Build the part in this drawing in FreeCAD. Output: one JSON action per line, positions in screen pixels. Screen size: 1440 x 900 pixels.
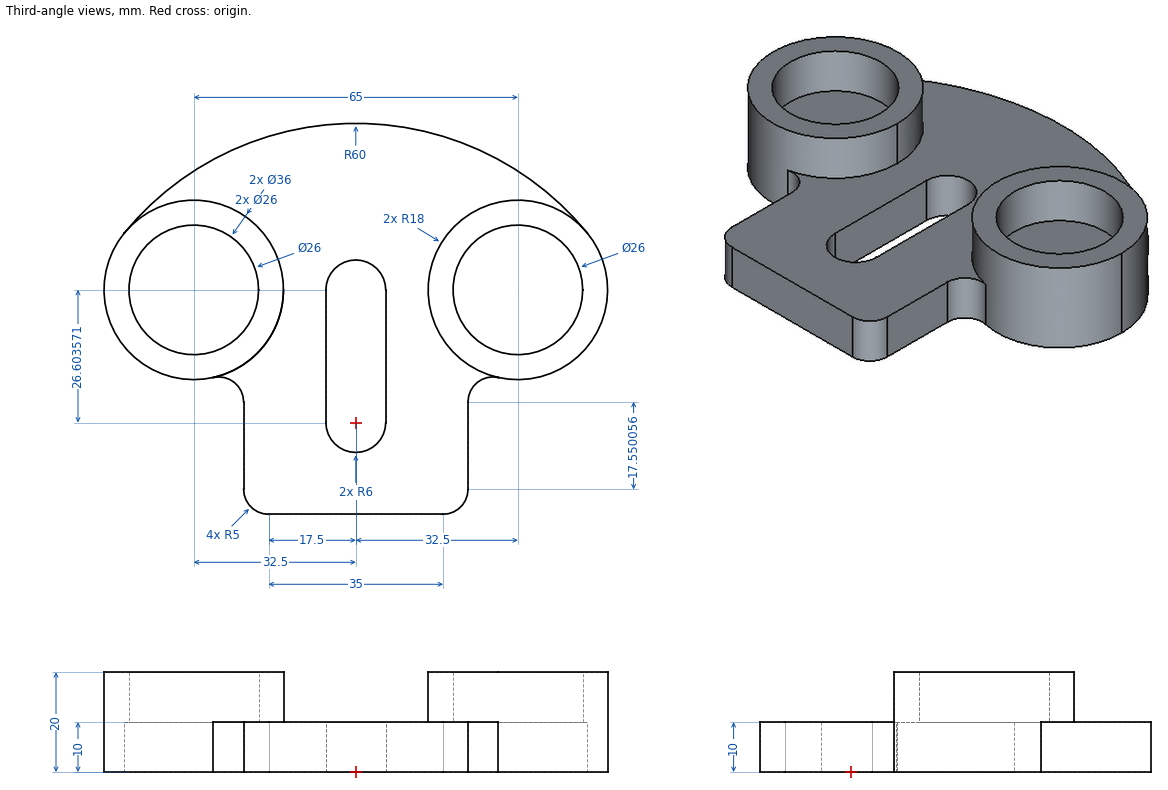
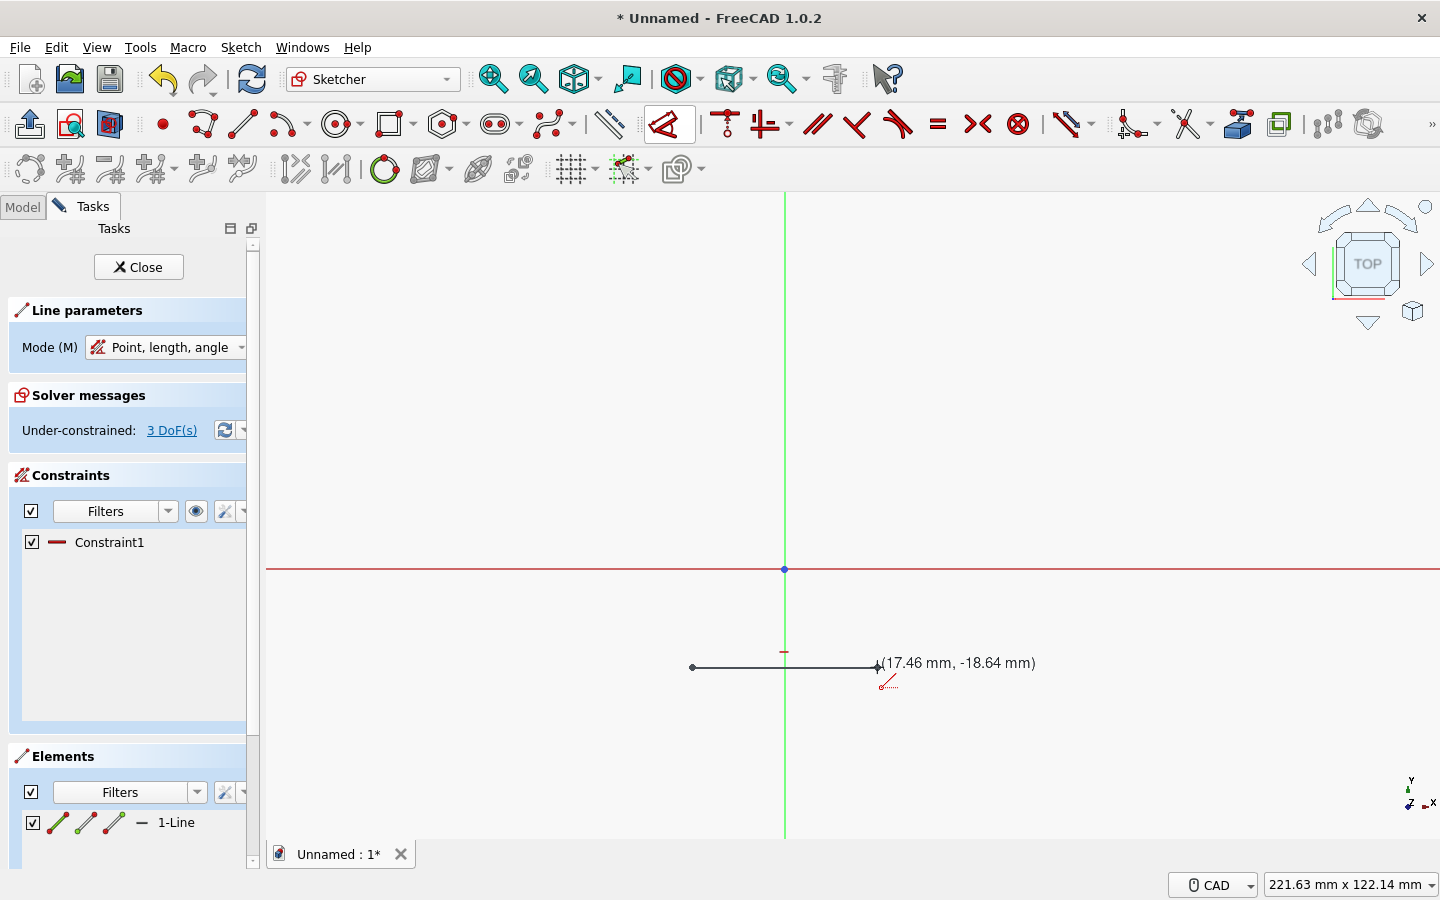
{"action": "left_click", "coordinate": [904, 640]}
{"action": "left_click", "coordinate": [904, 547]}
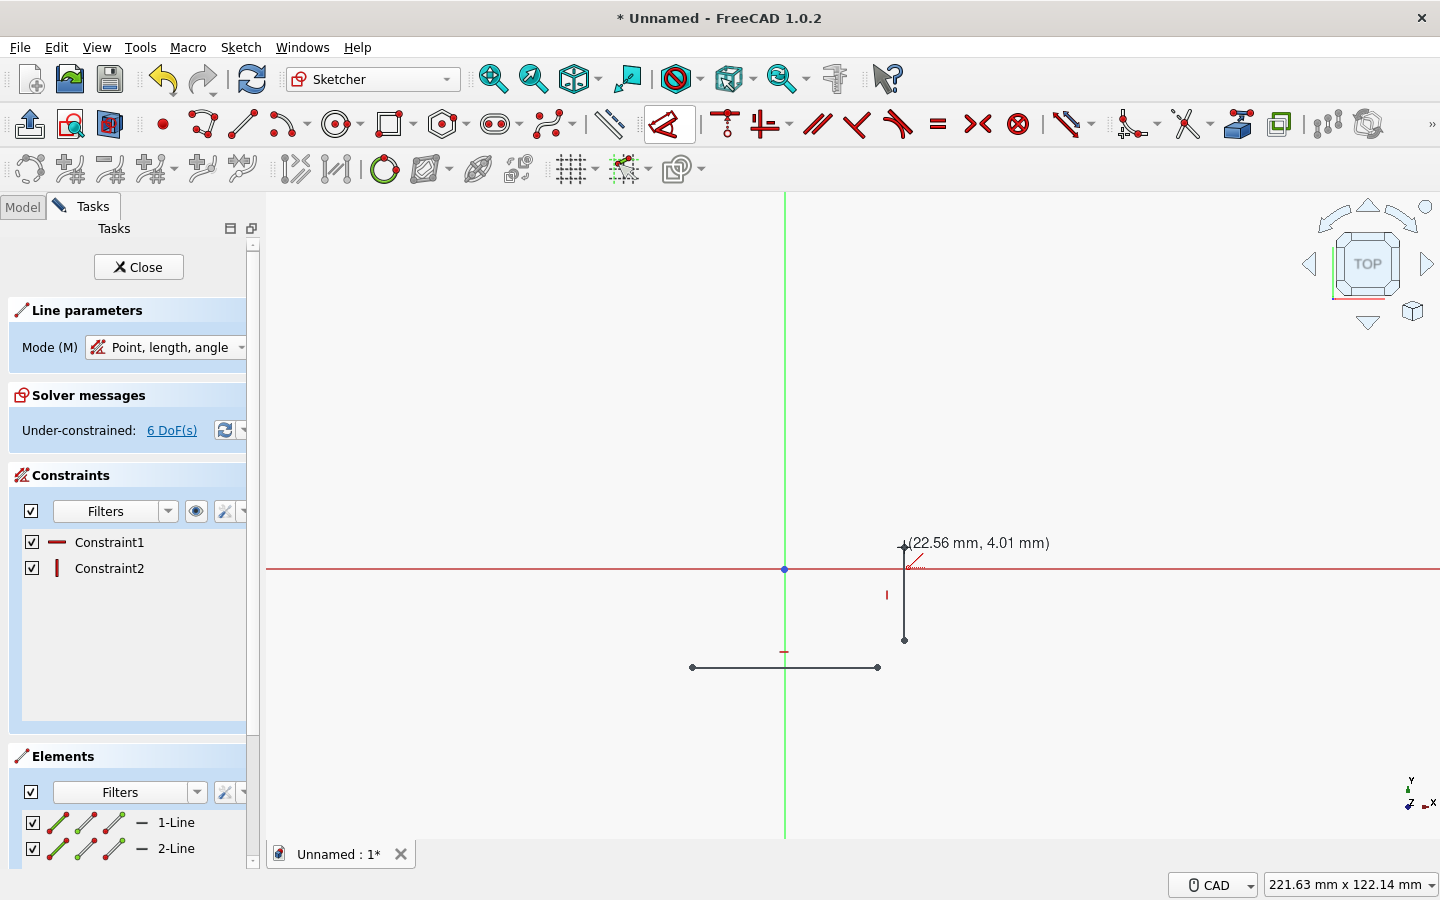
{"action": "left_click", "coordinate": [665, 547]}
{"action": "left_click", "coordinate": [665, 640]}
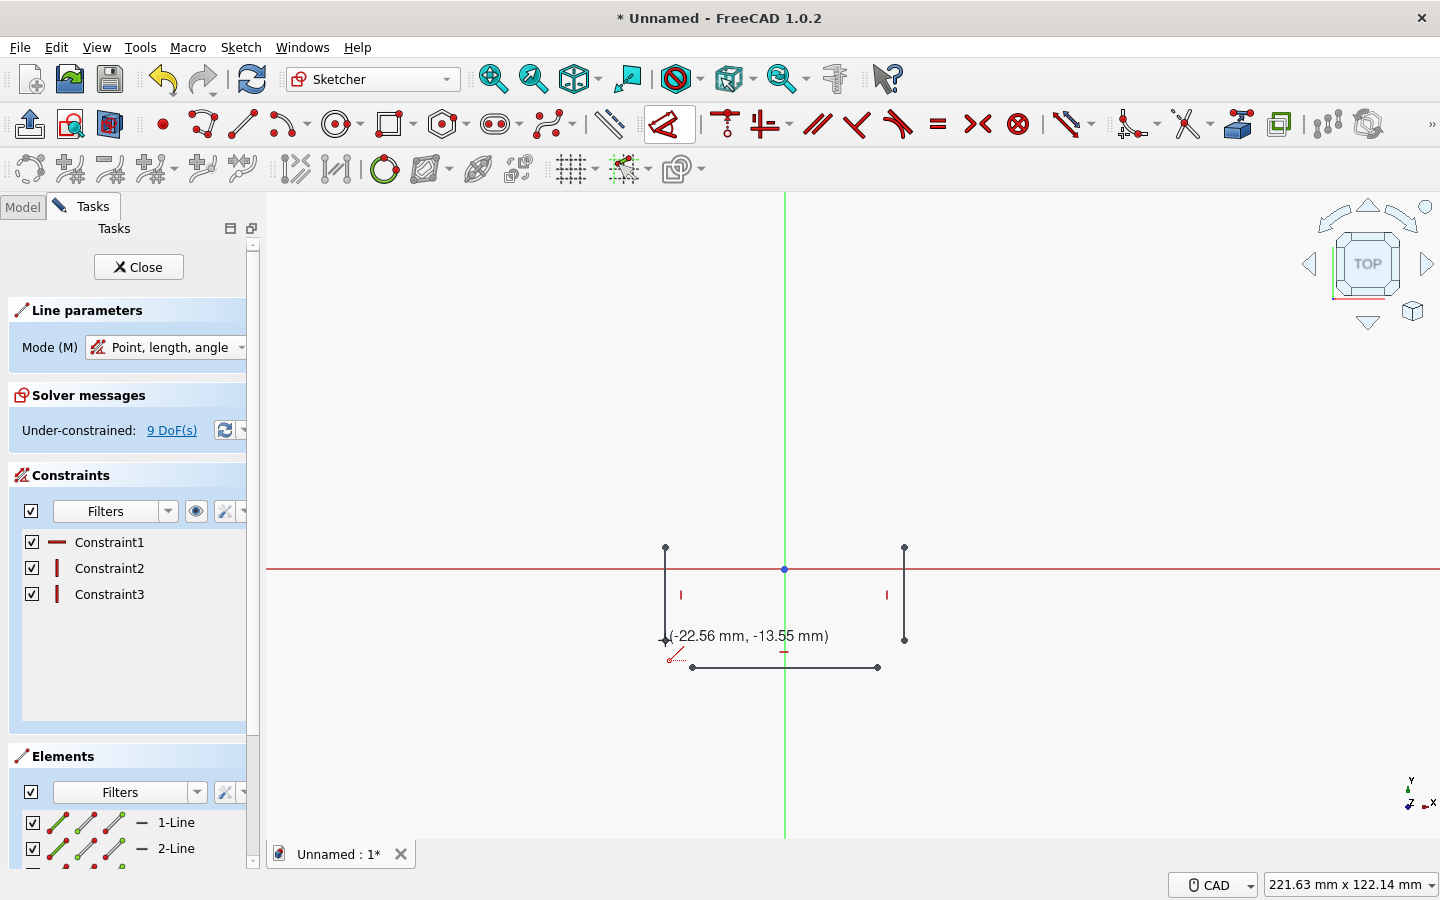
{"action": "left_click", "coordinate": [310, 124]}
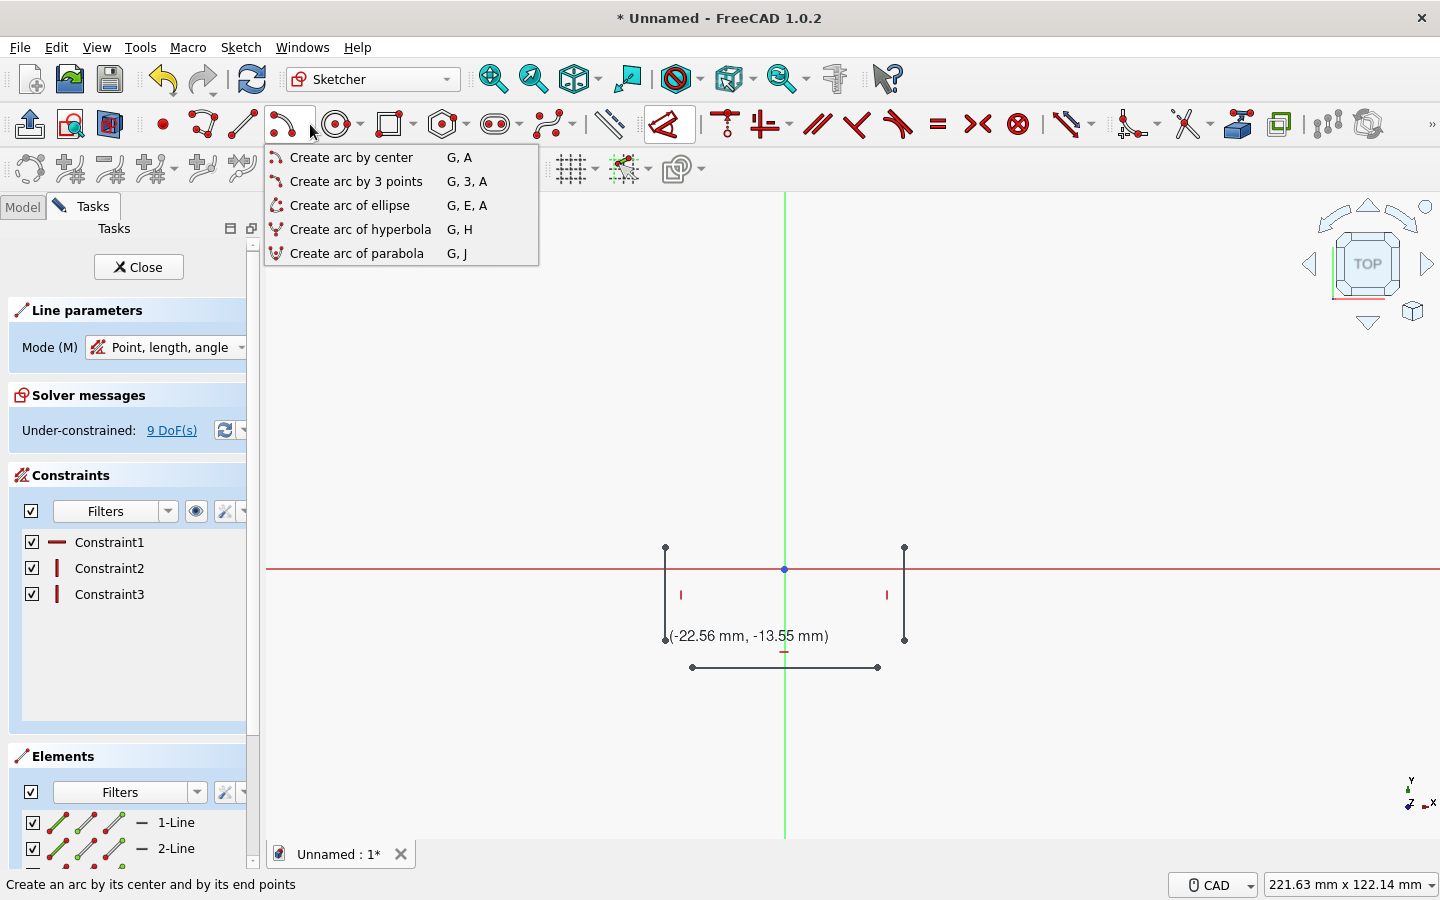
{"action": "left_click", "coordinate": [402, 181]}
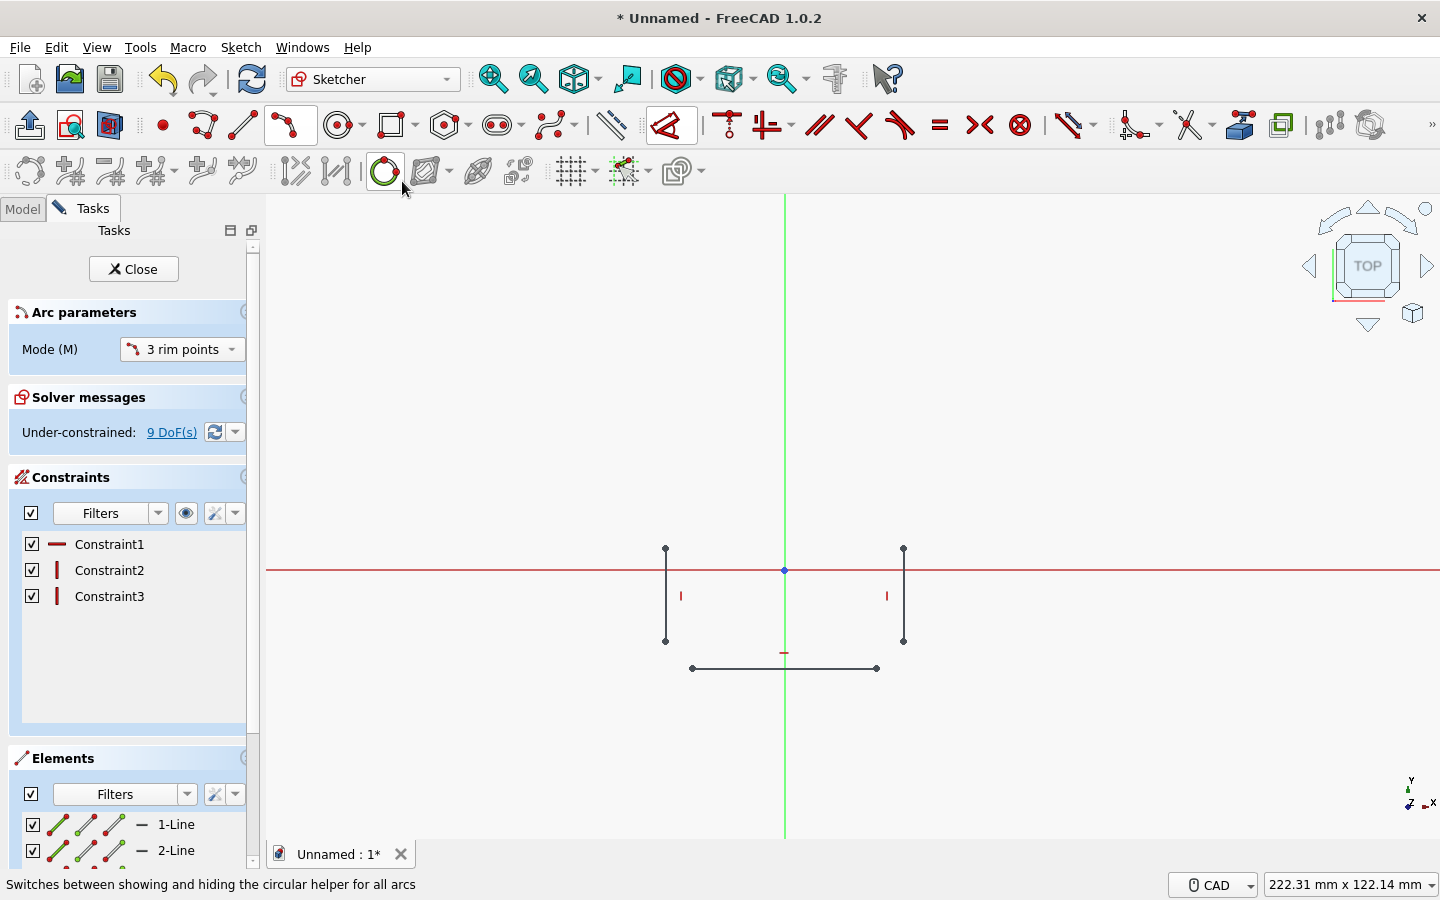
{"action": "left_click", "coordinate": [877, 669]}
{"action": "left_click", "coordinate": [904, 642]}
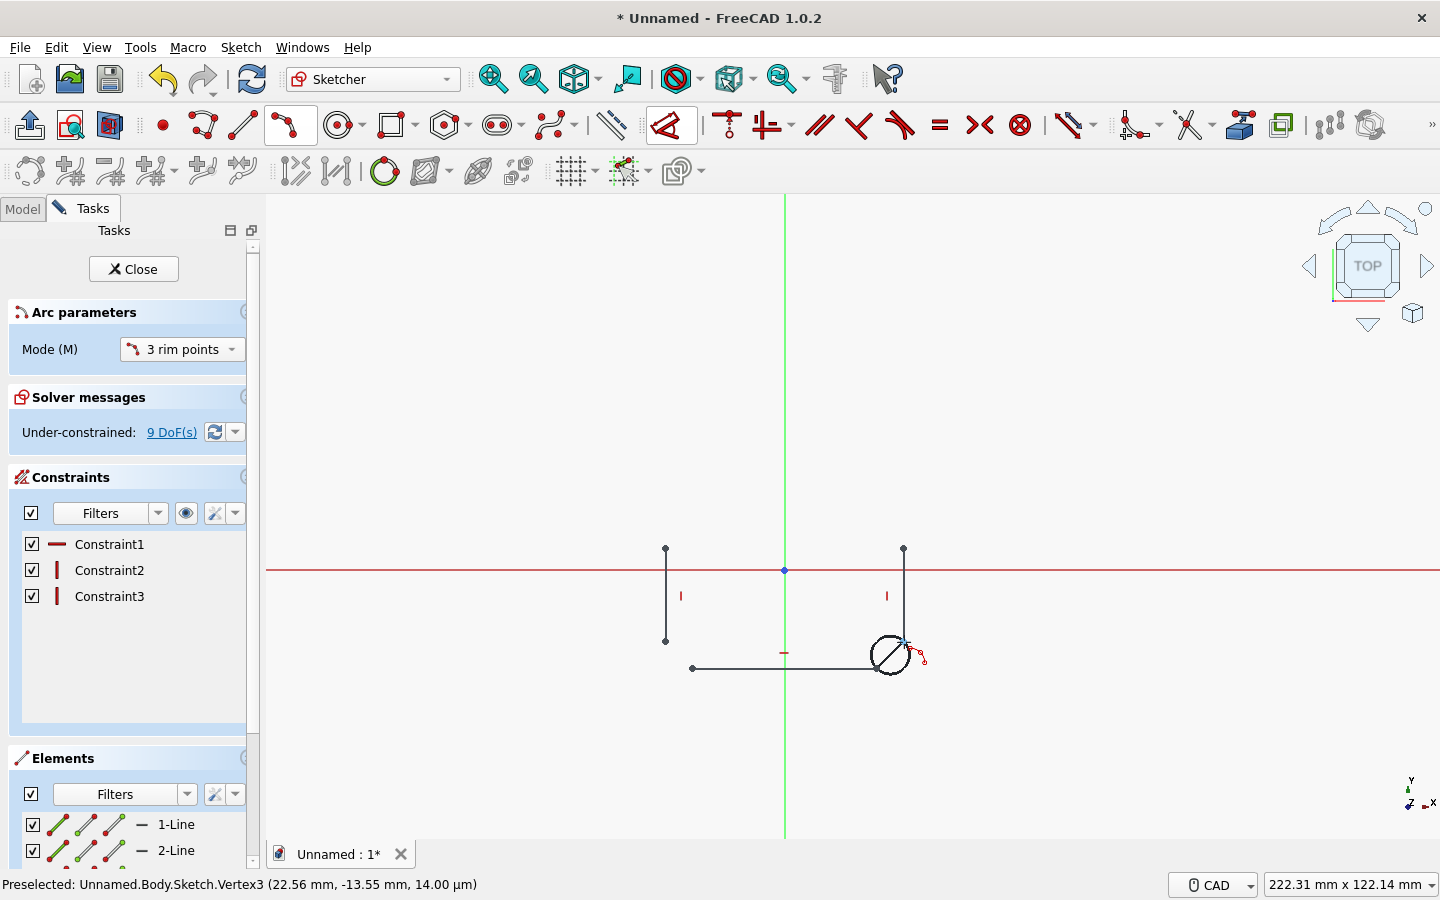
{"action": "scroll", "coordinate": [896, 659], "scroll_direction": "up", "scroll_amount": 4}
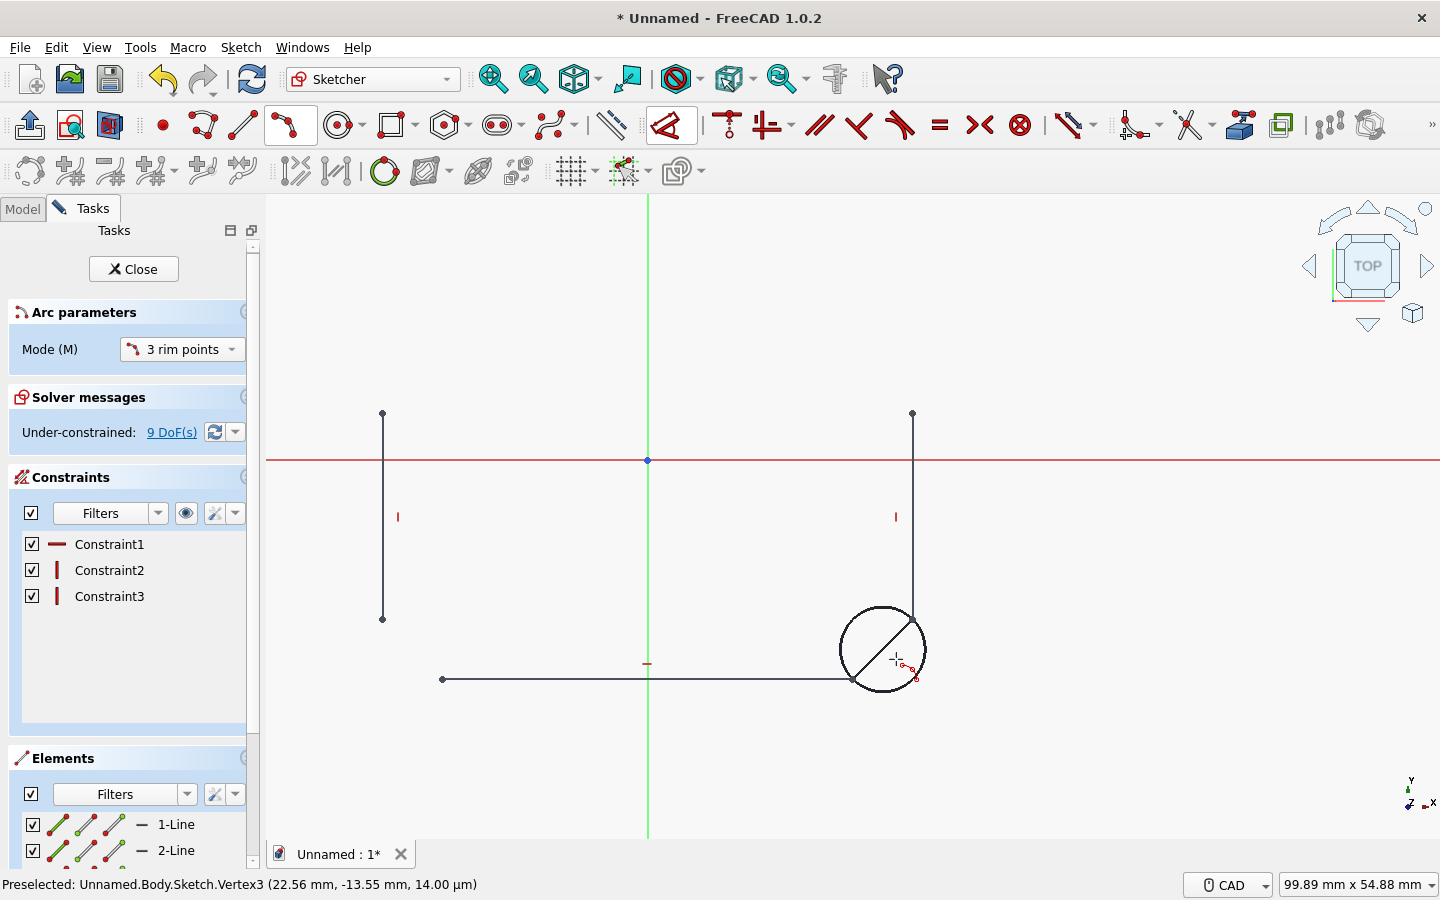
{"action": "left_click", "coordinate": [895, 659]}